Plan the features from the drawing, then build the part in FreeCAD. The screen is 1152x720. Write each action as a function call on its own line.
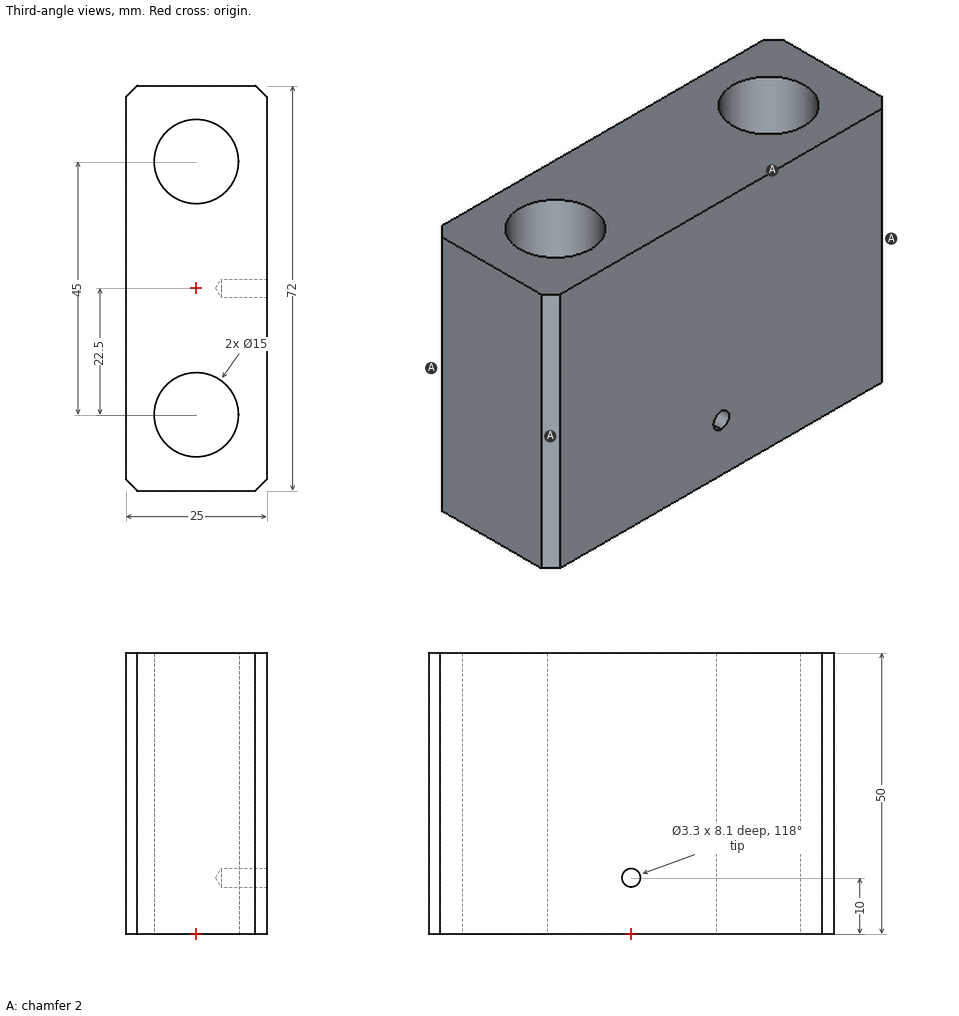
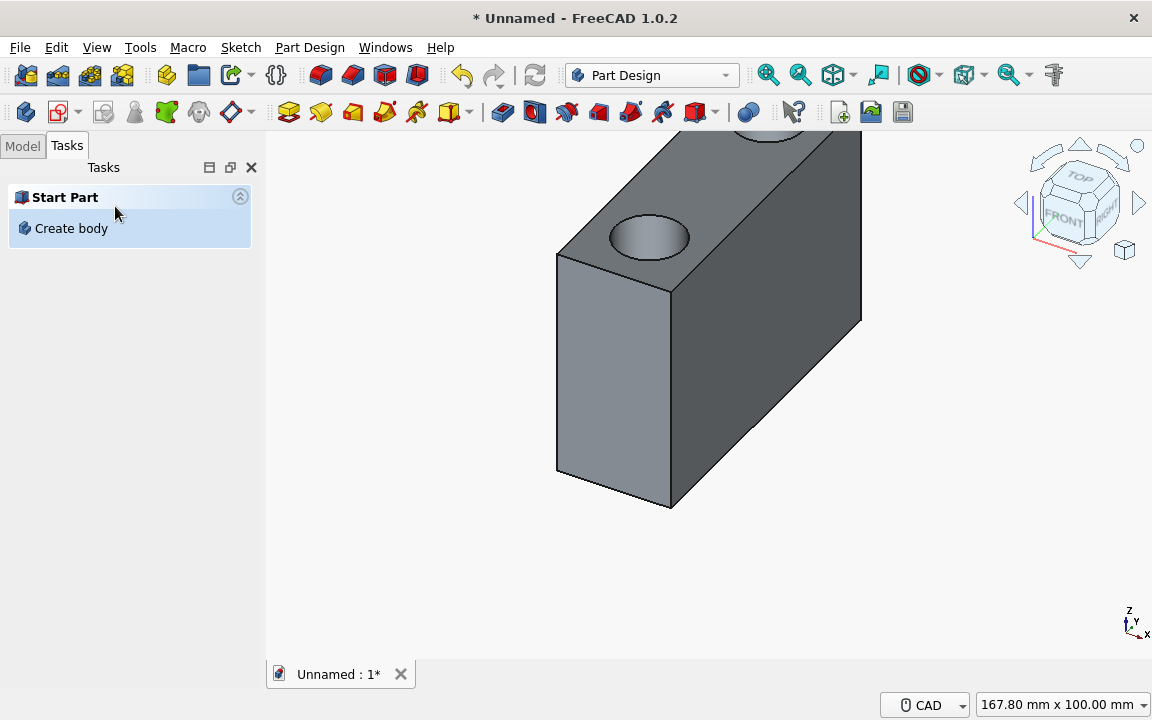
key(v)
key(f)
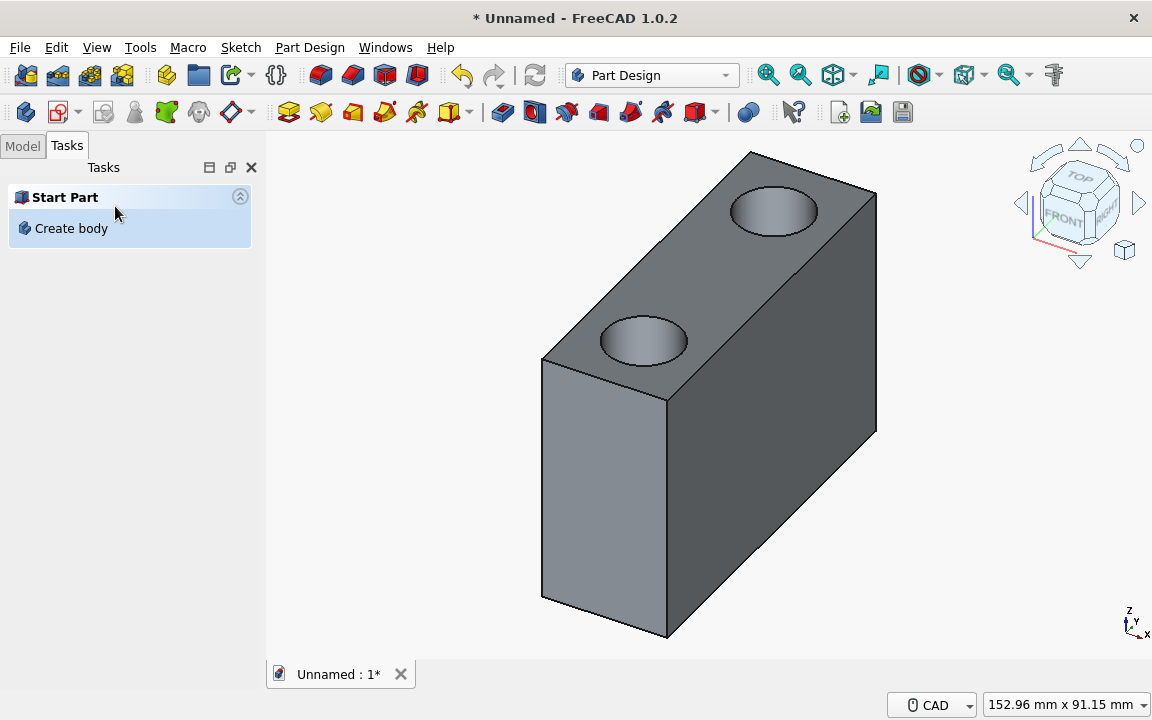
click(801, 385)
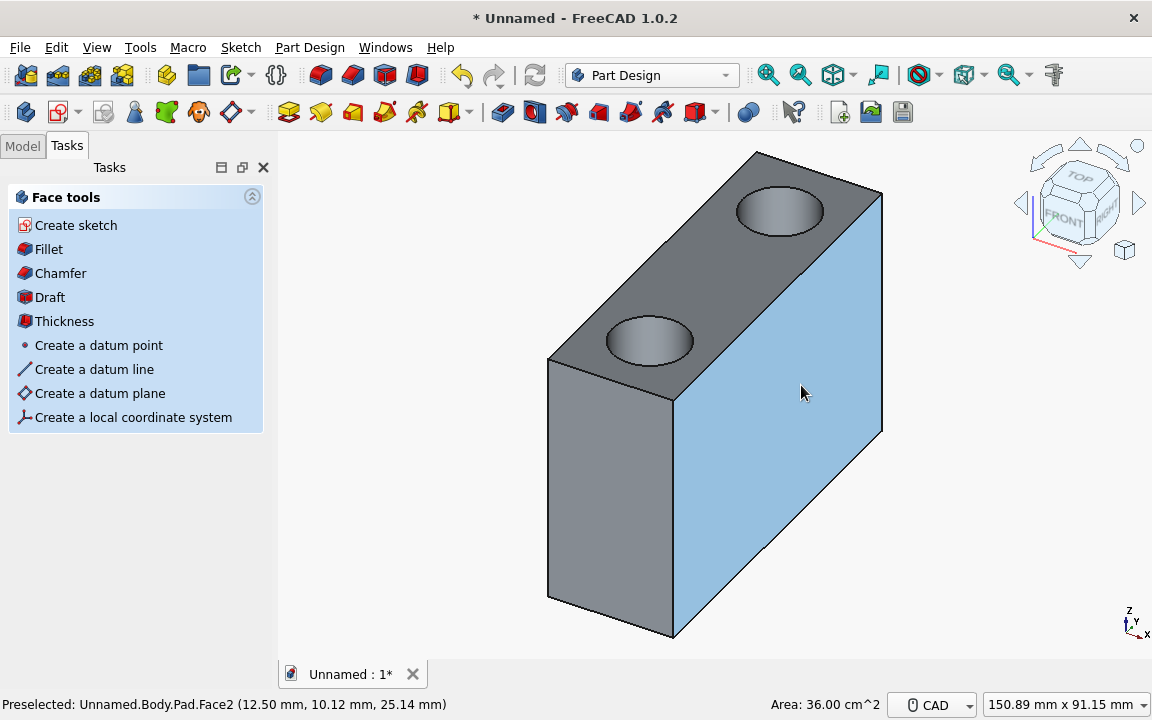
click(58, 112)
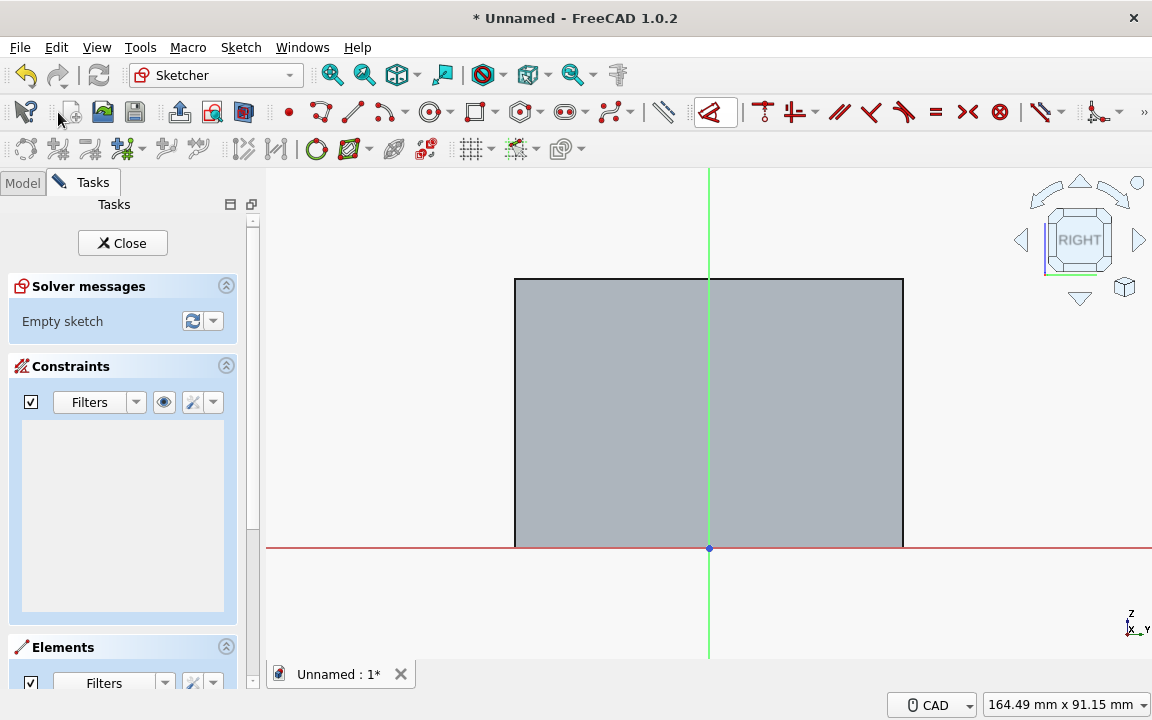
scroll(713, 500, up, 14)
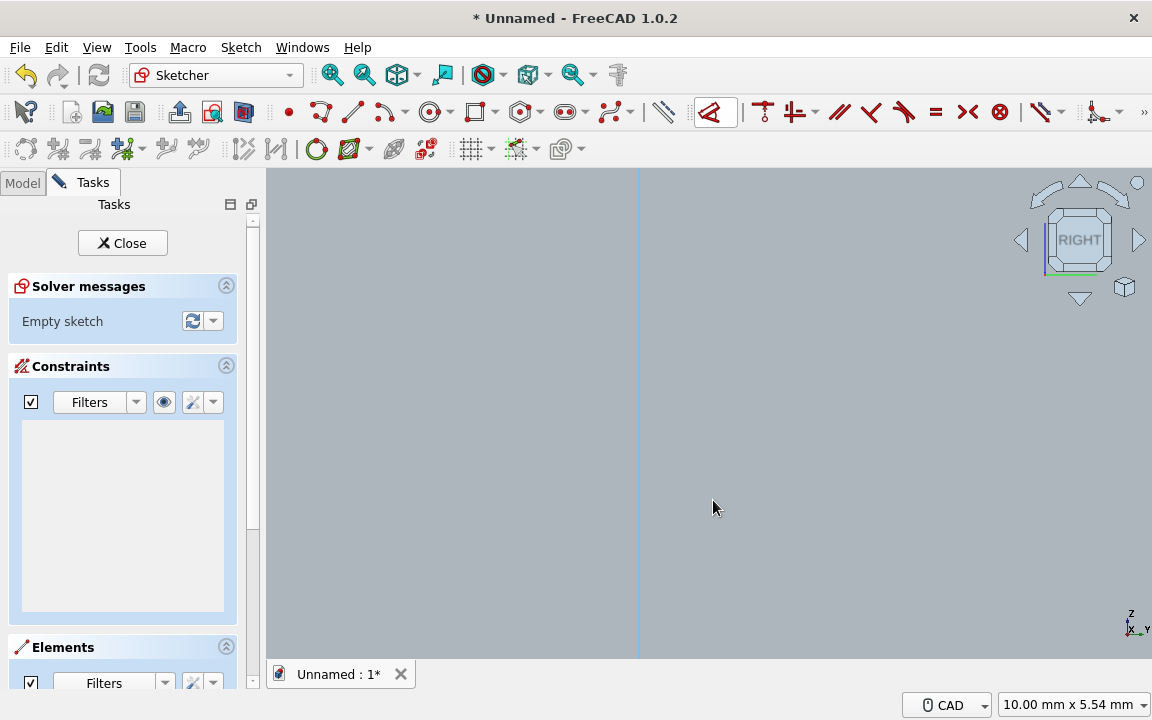
key(g)
key(c)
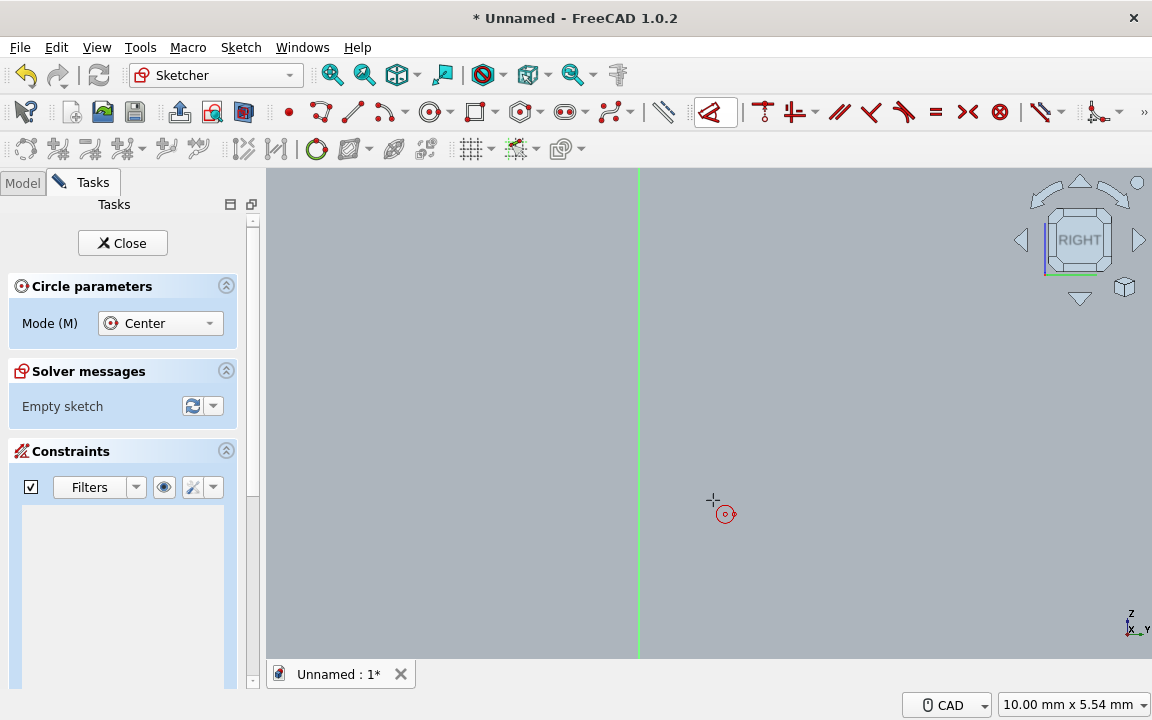
click(639, 396)
move(743, 292)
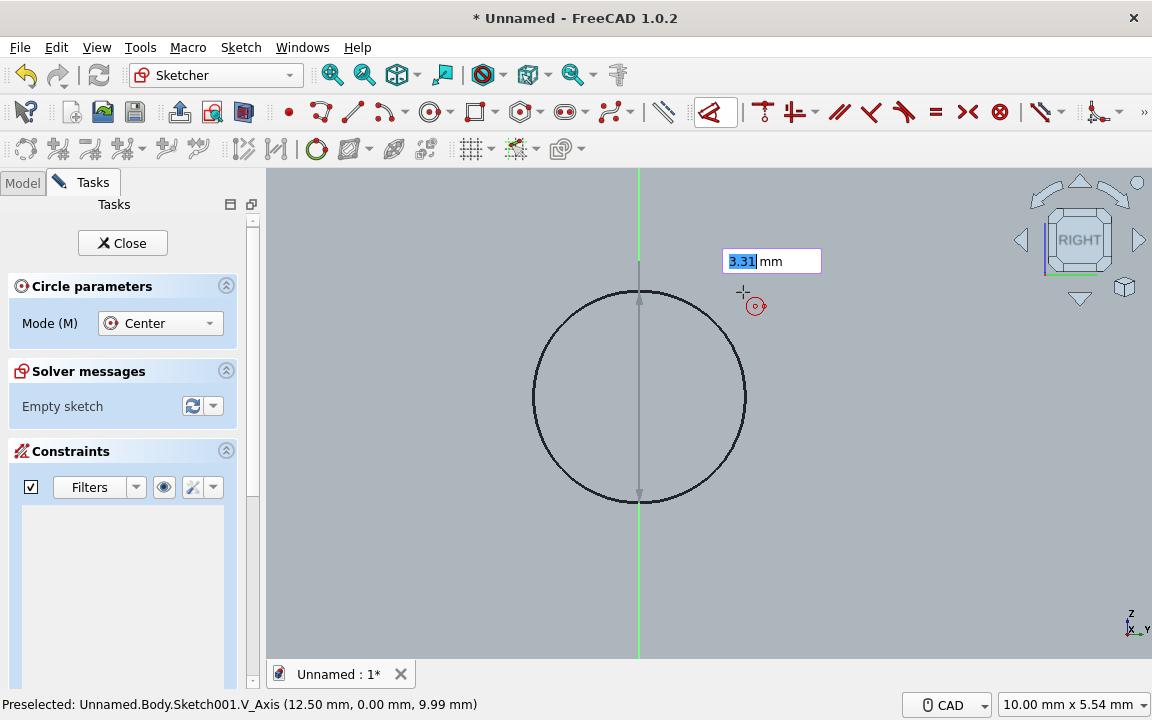
text(3.3)
key(Return)
key(Escape)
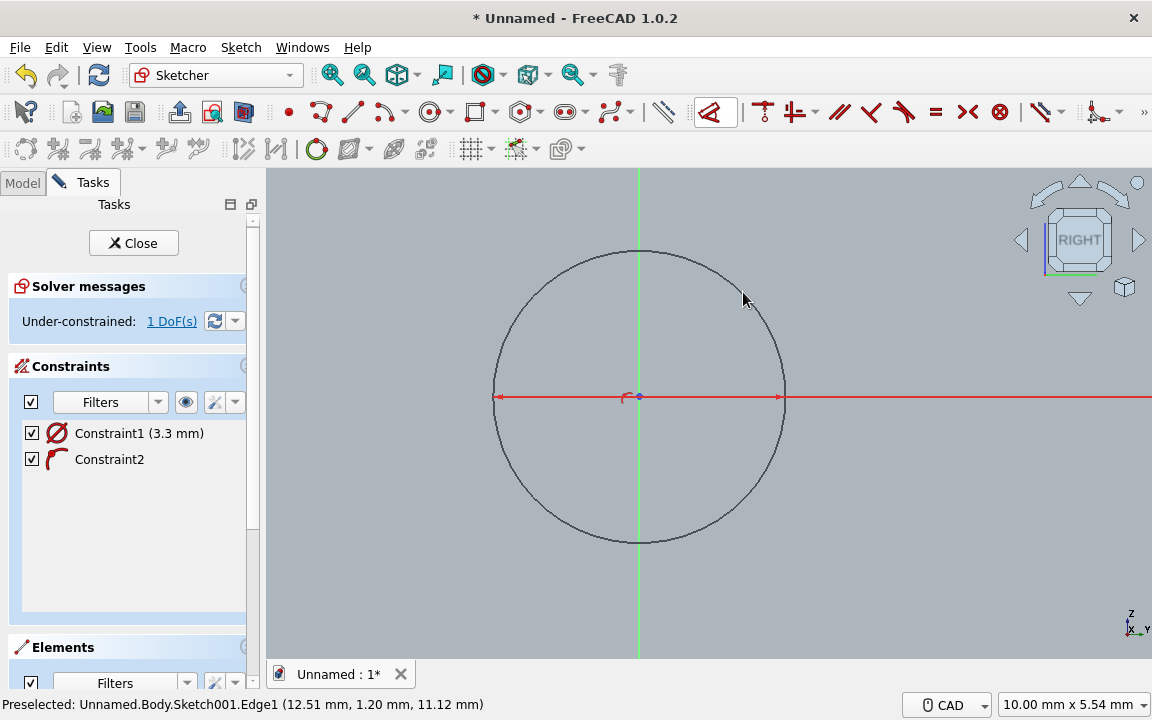
click(639, 397)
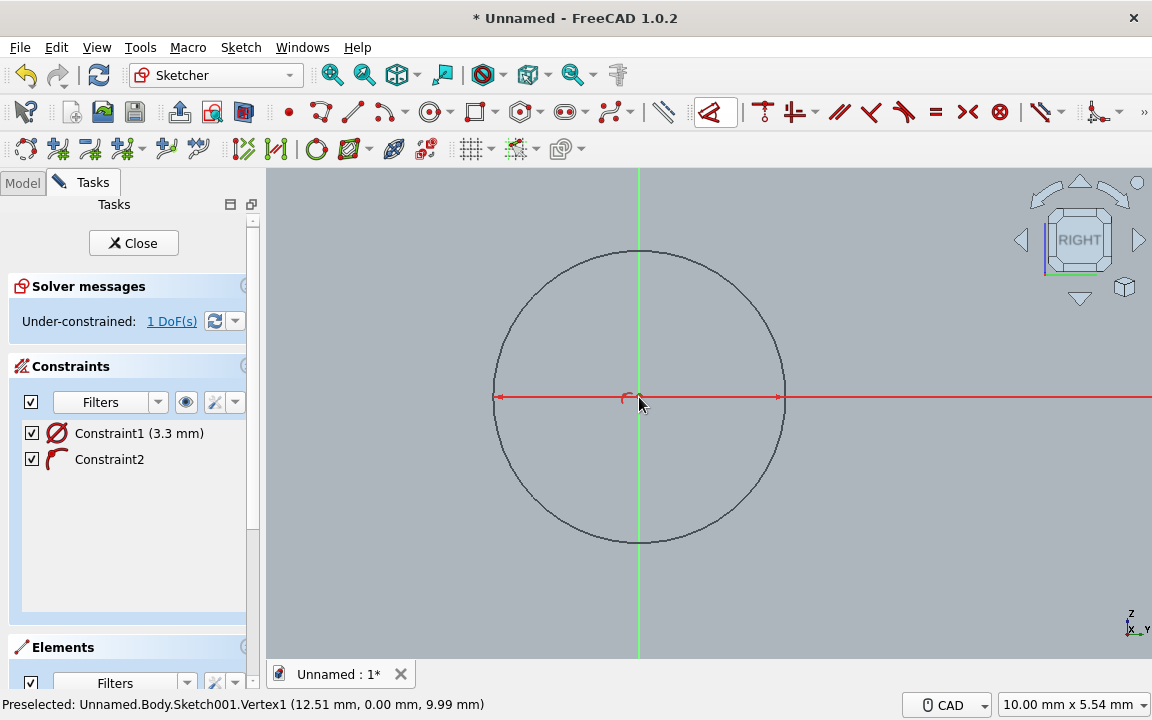
key(i)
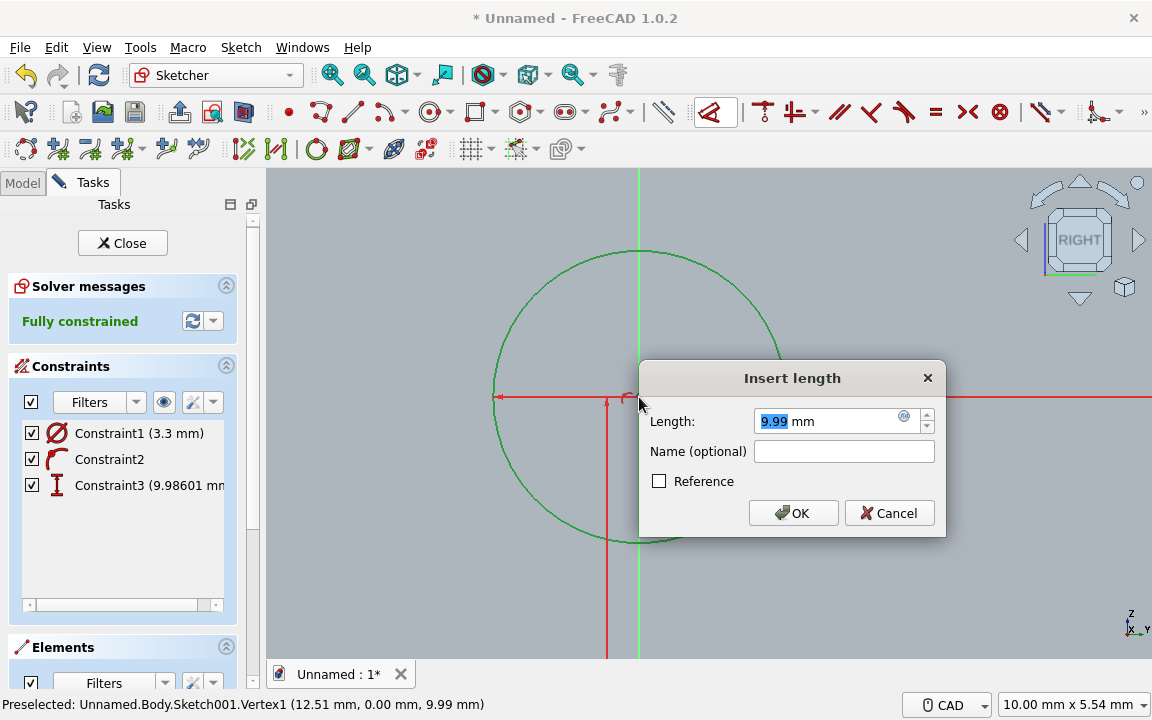
text(10)
key(Return)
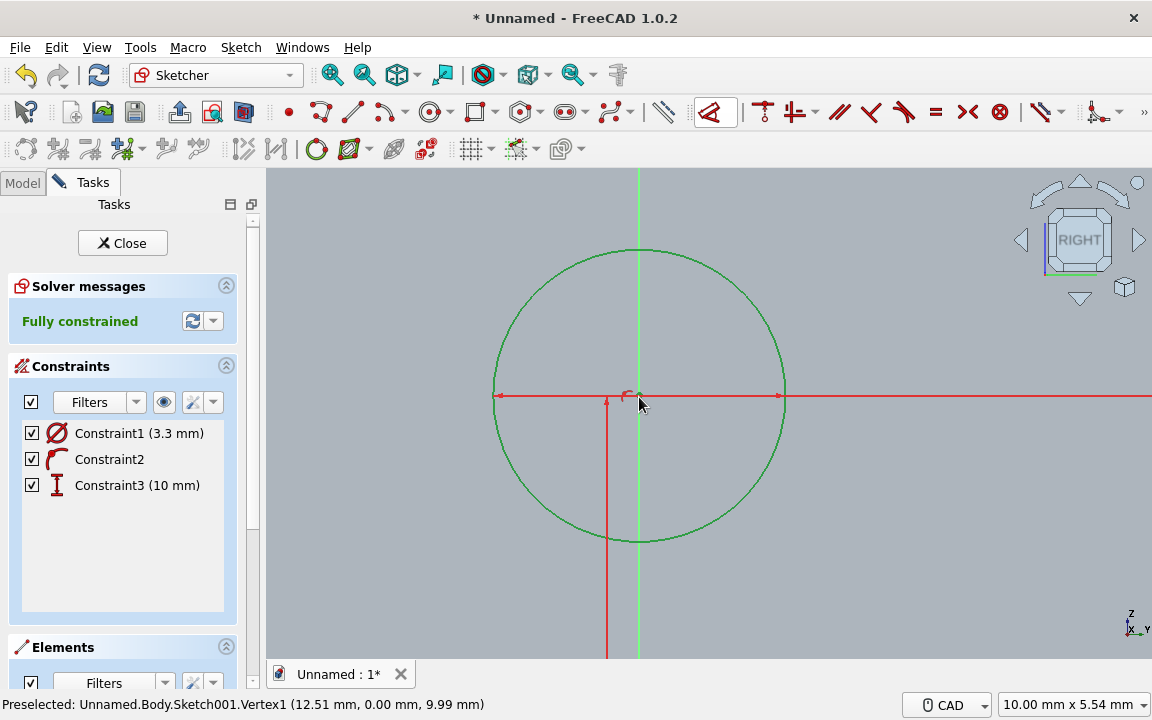
click(123, 243)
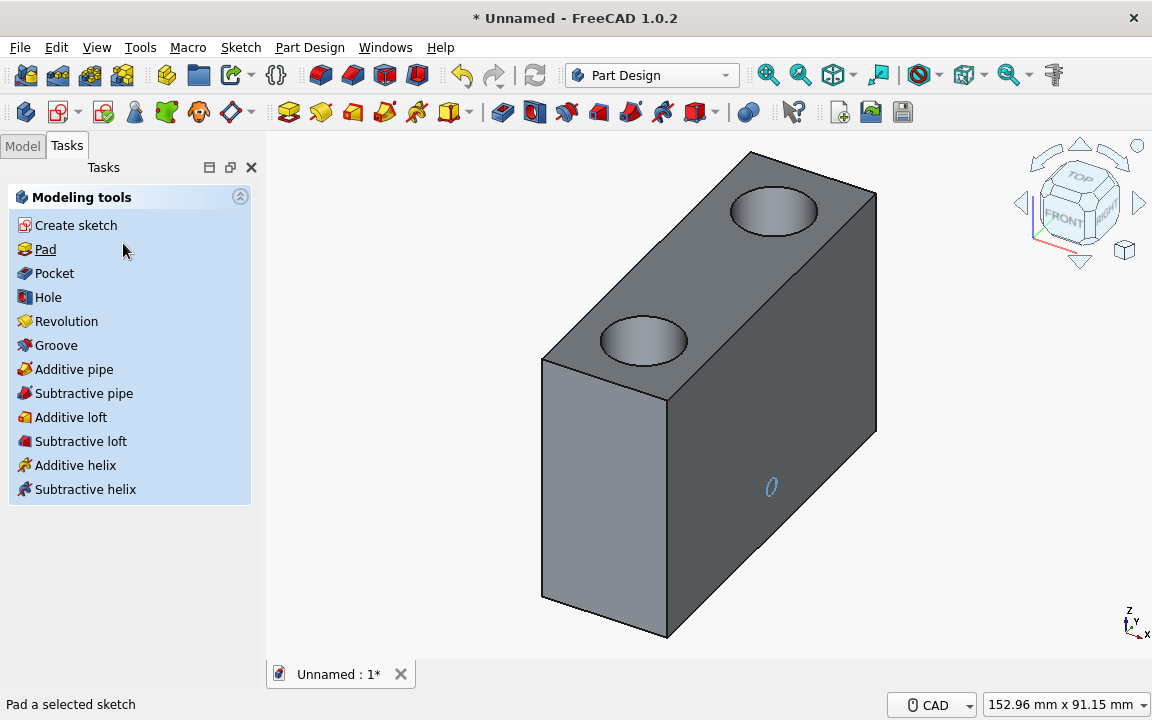
click(536, 112)